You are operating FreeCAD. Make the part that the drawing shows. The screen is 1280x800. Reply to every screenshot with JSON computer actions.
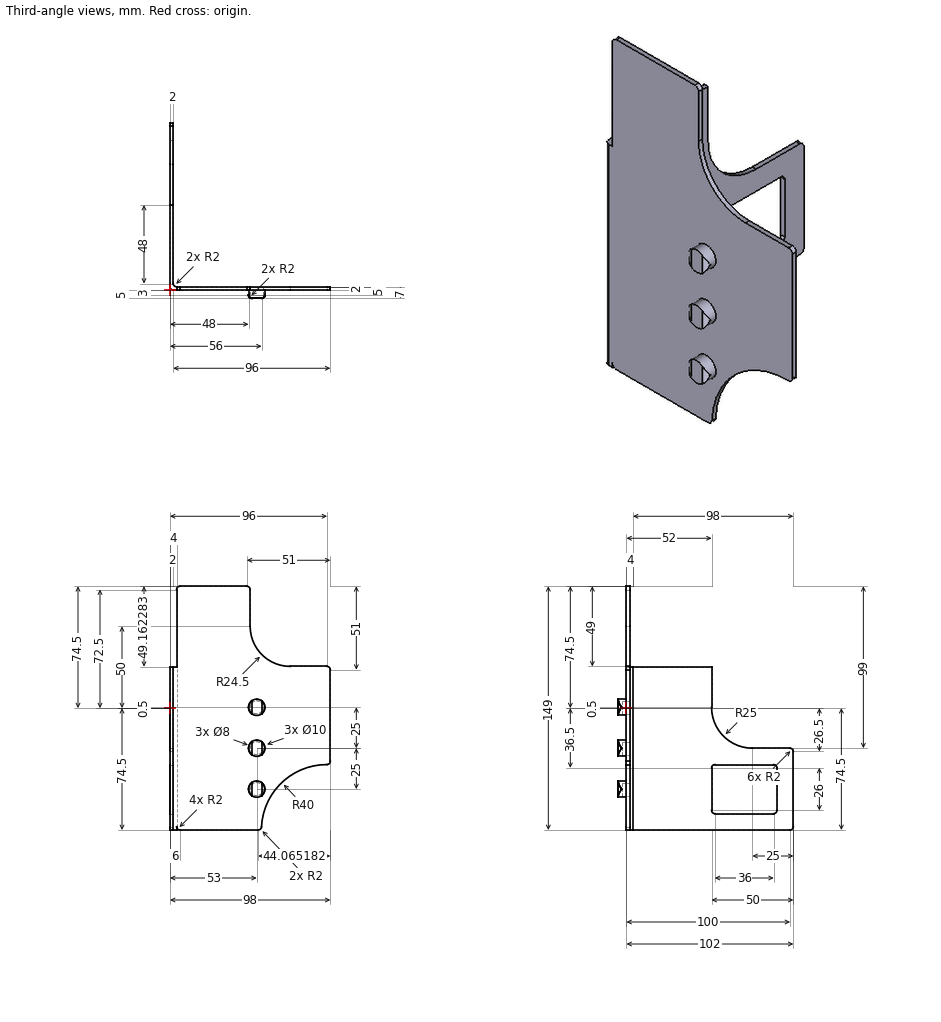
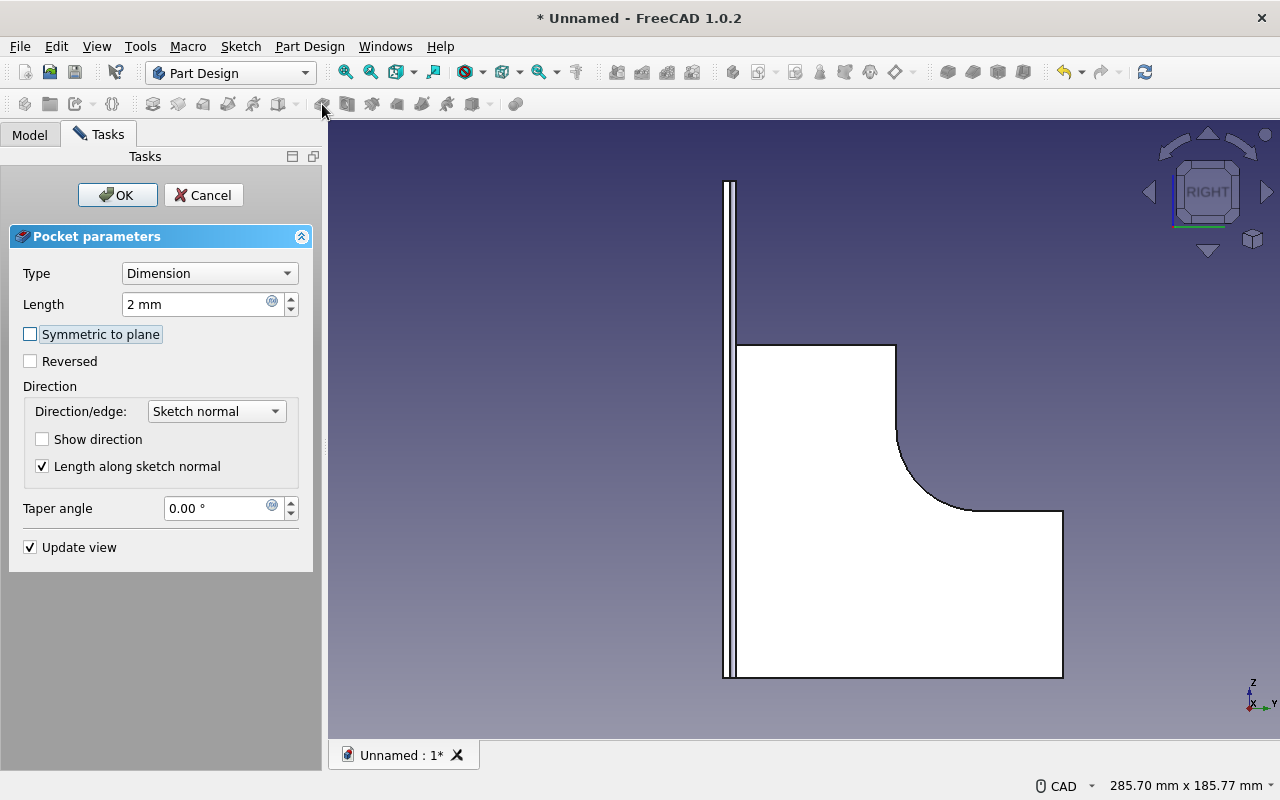
{"action": "left_click", "coordinate": [118, 195]}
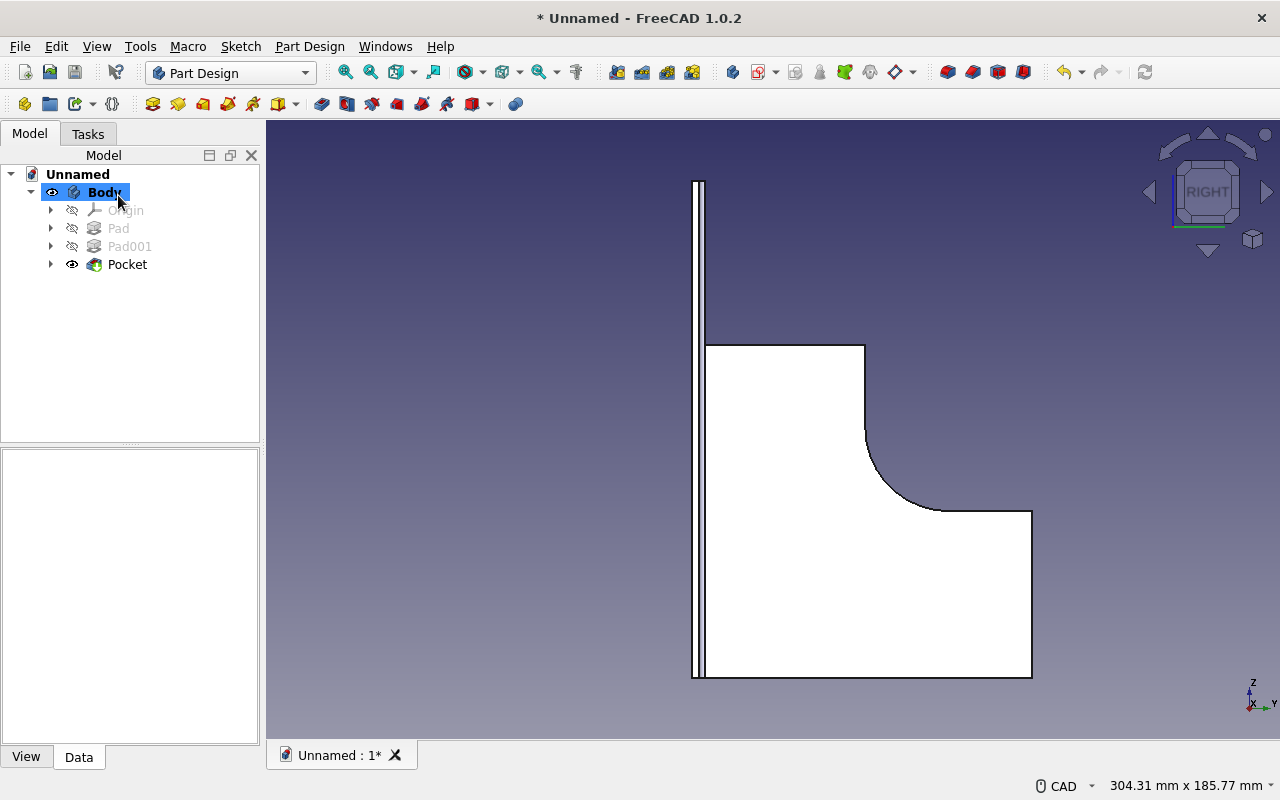
{"action": "key", "text": "4"}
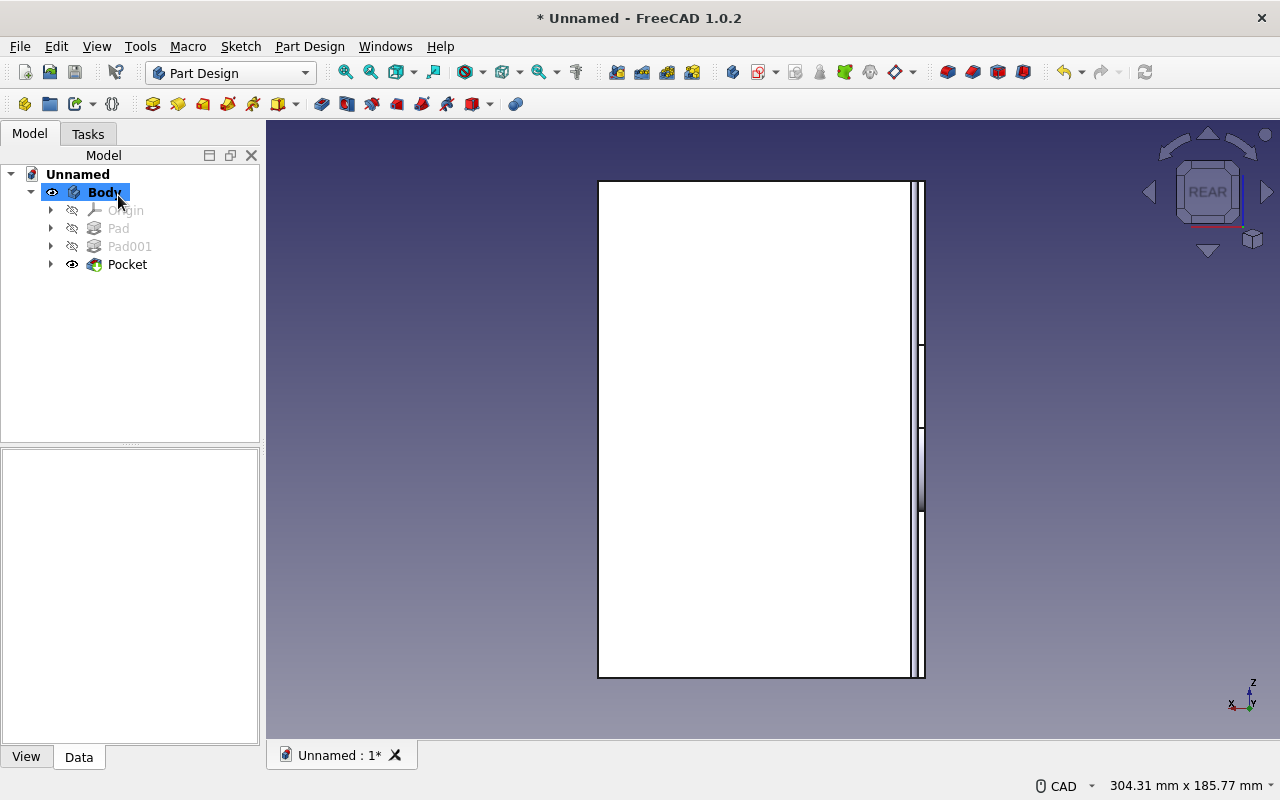
{"action": "left_click", "coordinate": [755, 358]}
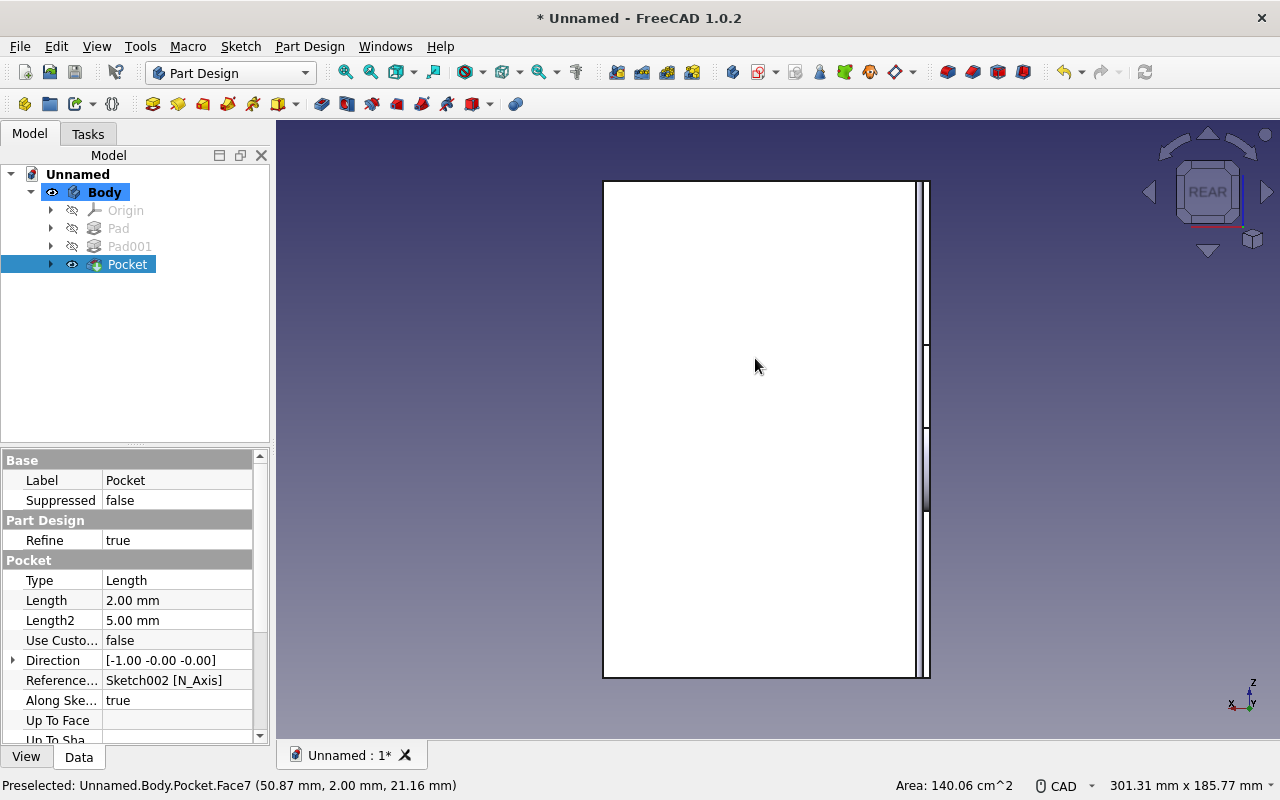
{"action": "left_click", "coordinate": [758, 72]}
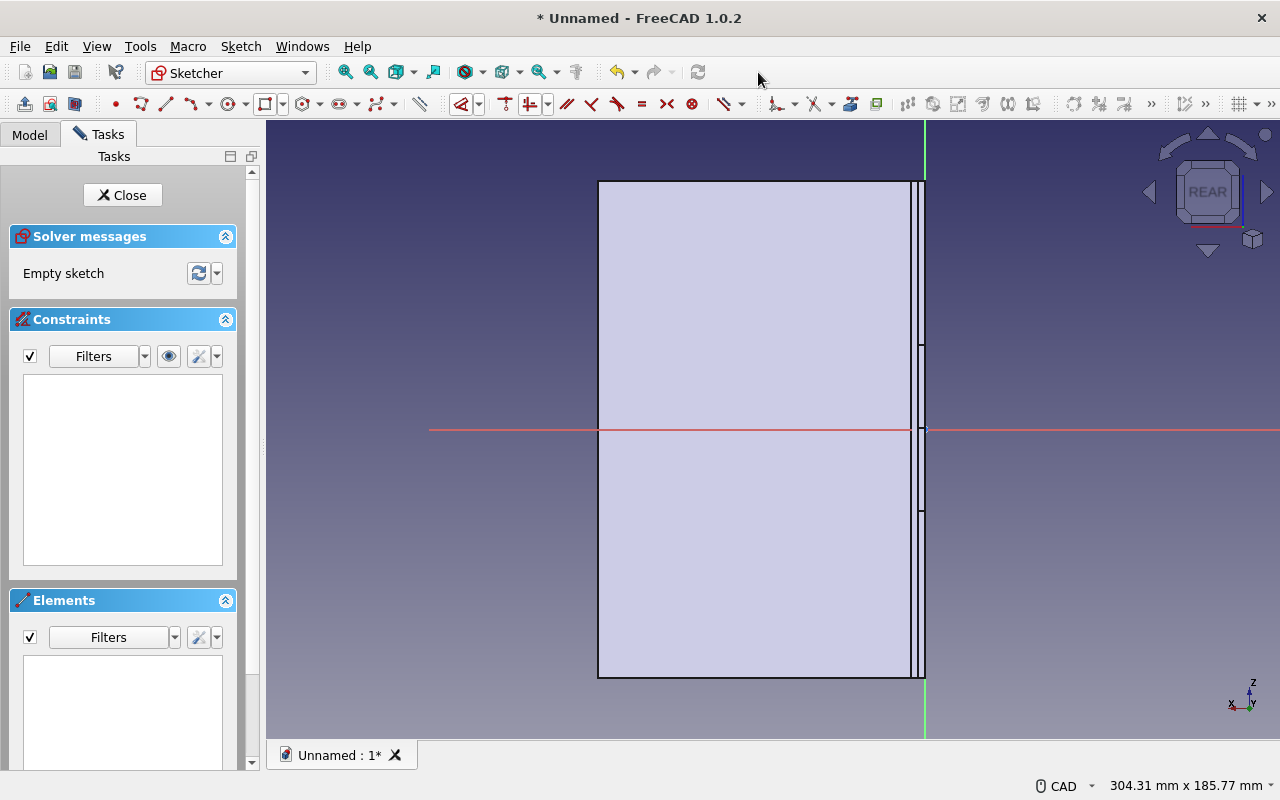
{"action": "scroll", "coordinate": [1115, 148], "scroll_direction": "up", "scroll_amount": 2}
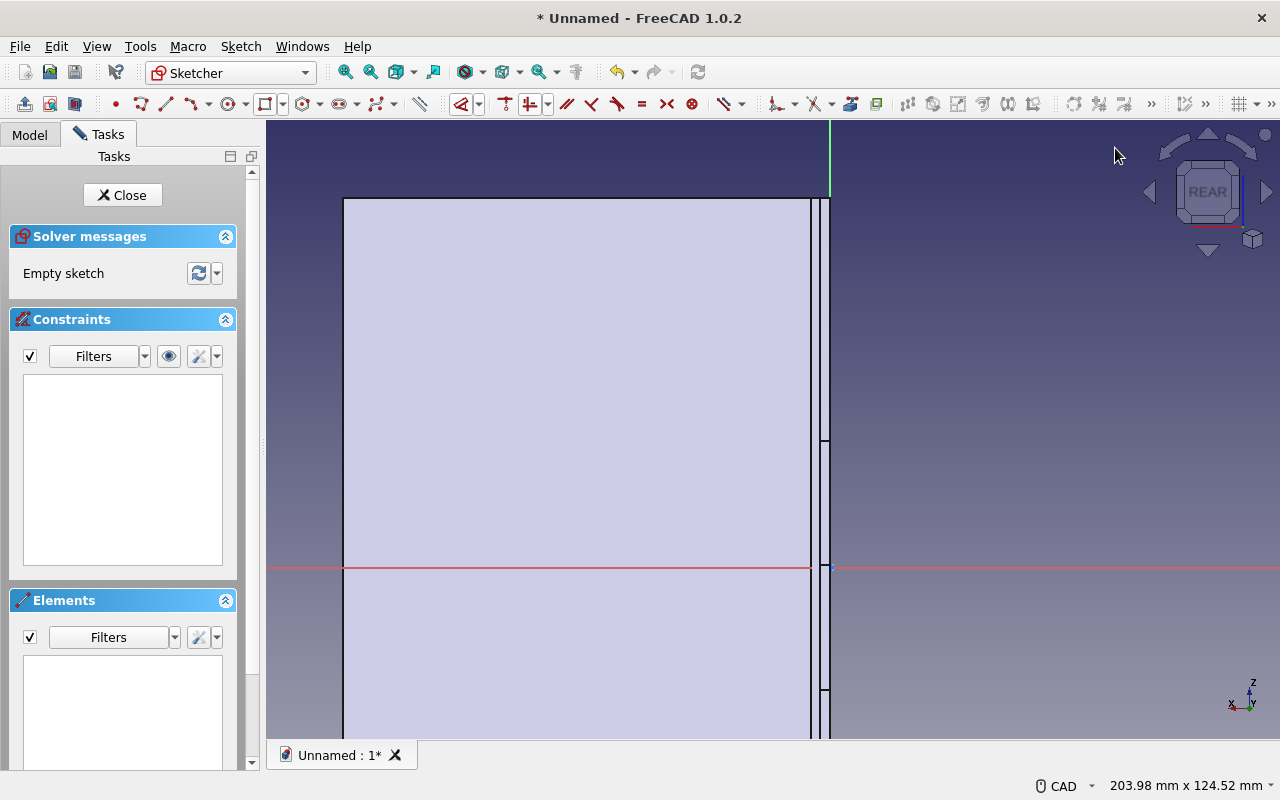
{"action": "key", "text": "g r"}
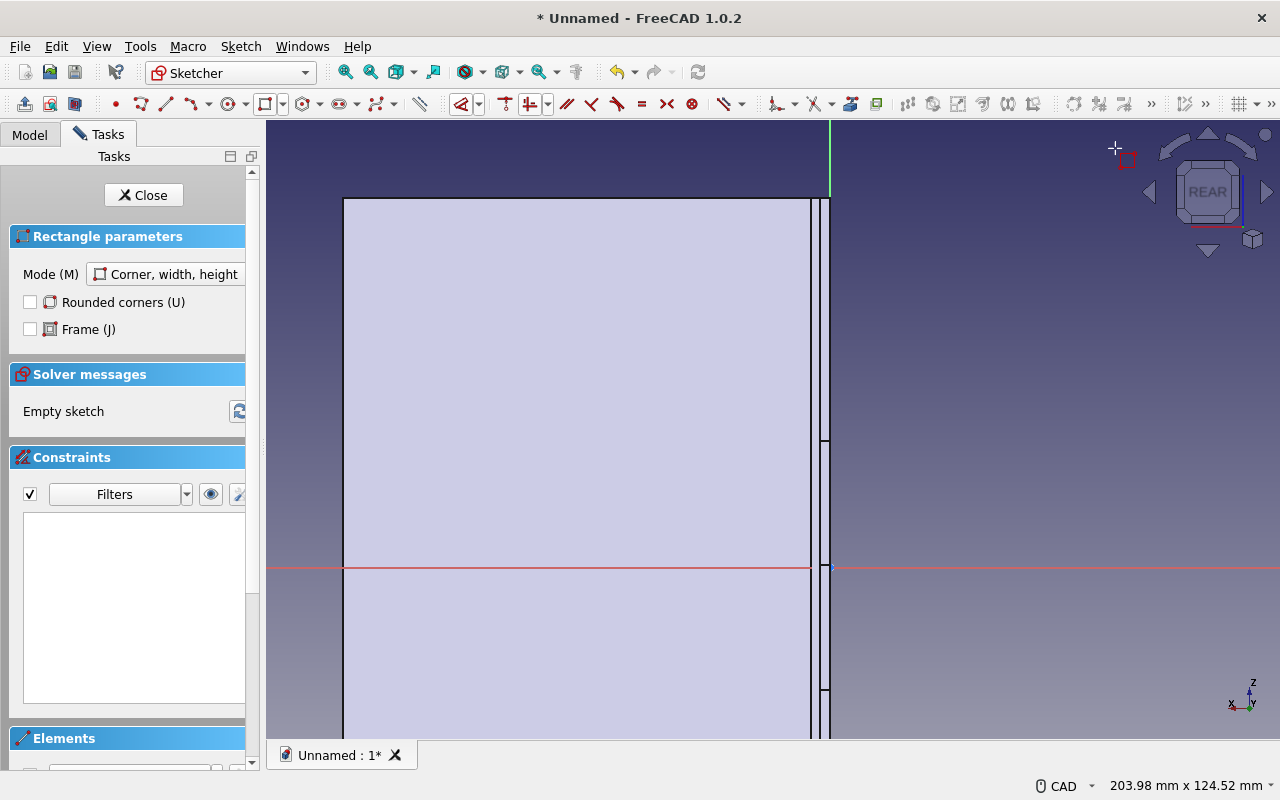
{"action": "left_click", "coordinate": [811, 198]}
{"action": "left_click", "coordinate": [830, 442]}
{"action": "key", "text": "Escape"}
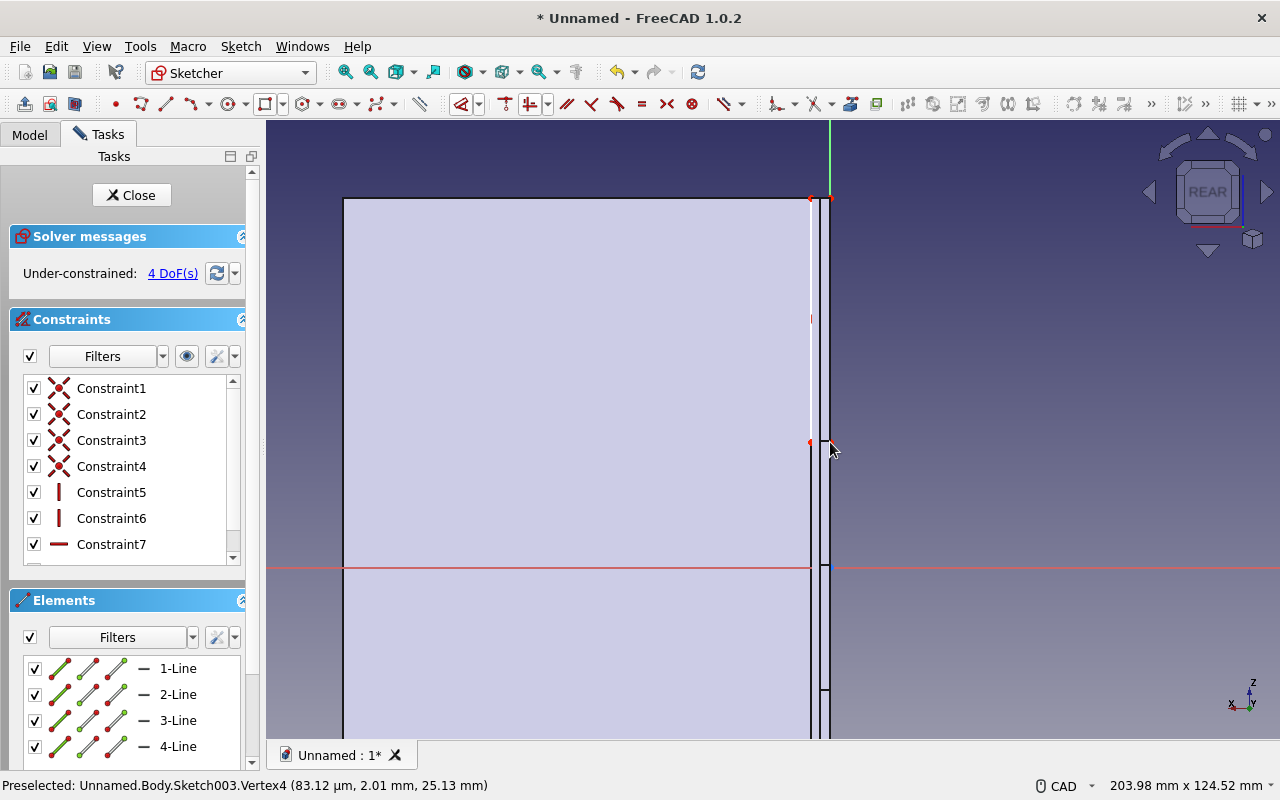
{"action": "left_click", "coordinate": [830, 443]}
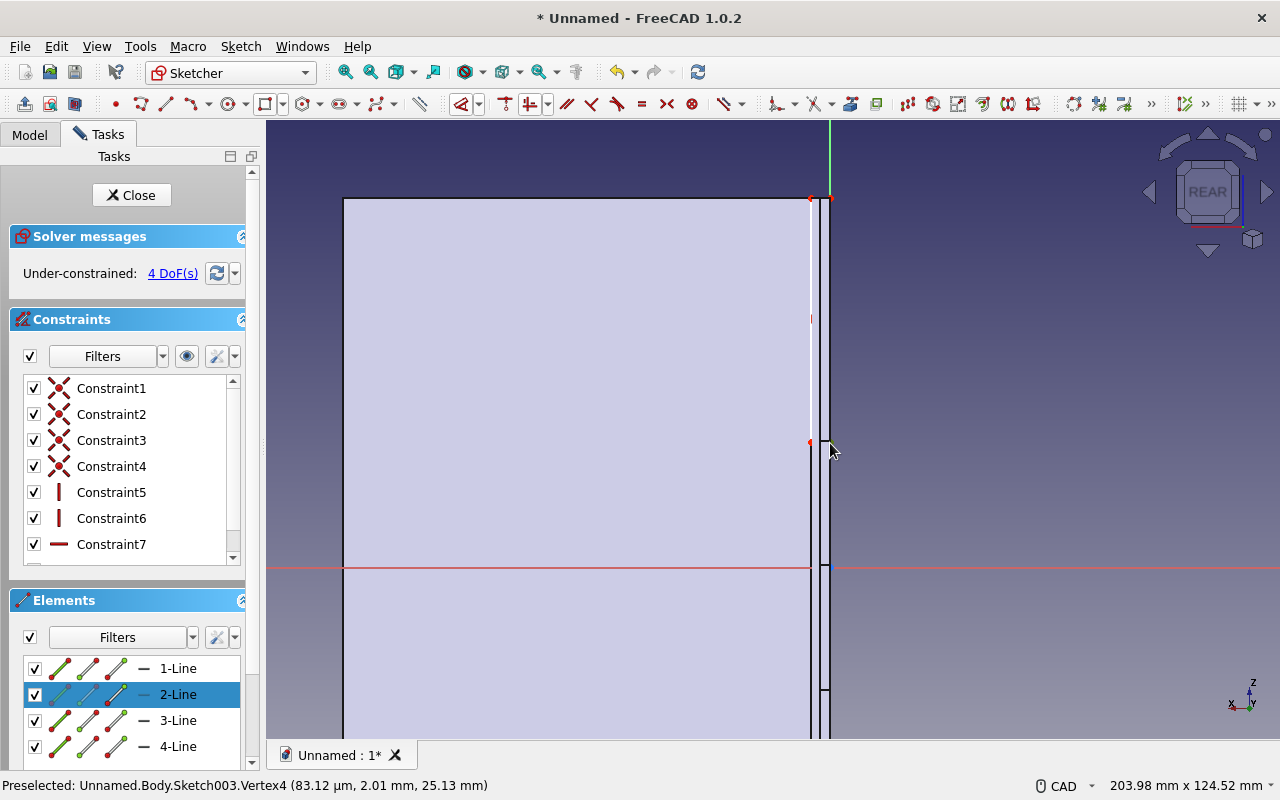
{"action": "left_click", "coordinate": [830, 671]}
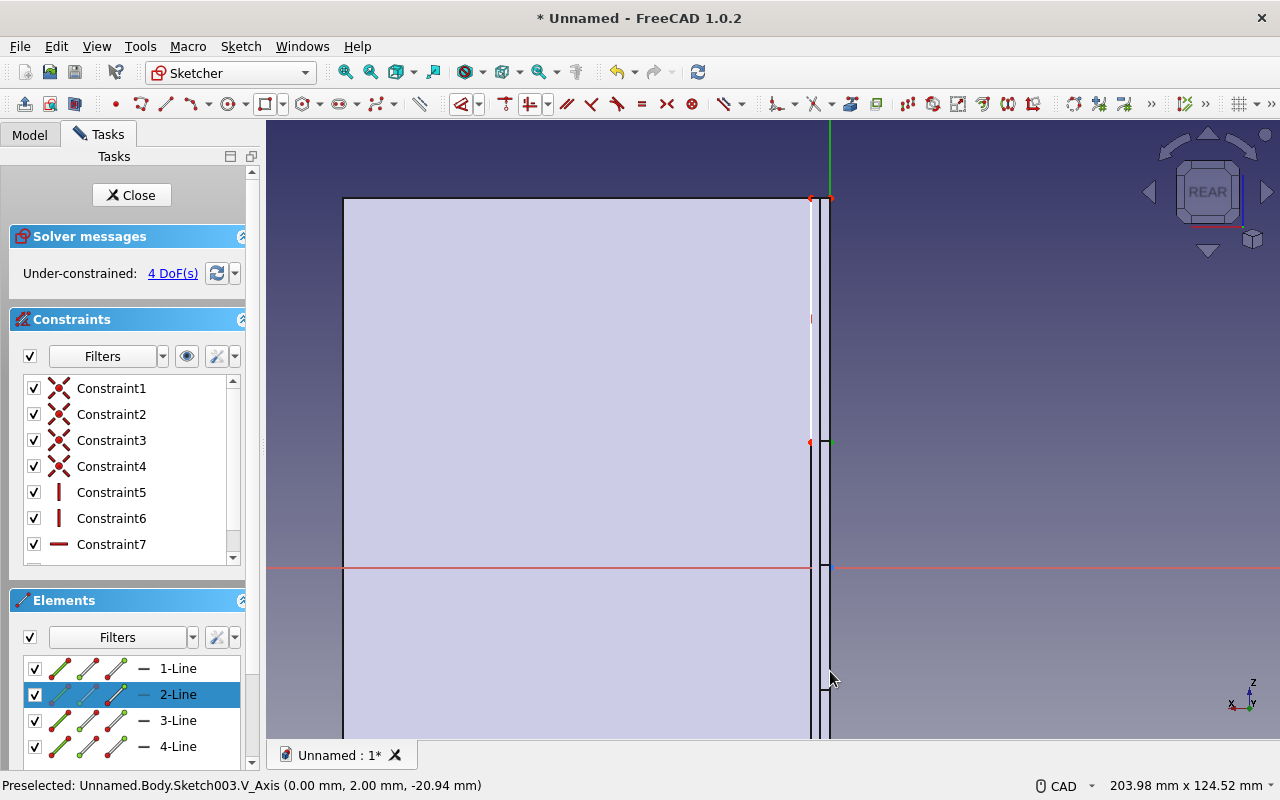
{"action": "key", "text": "c"}